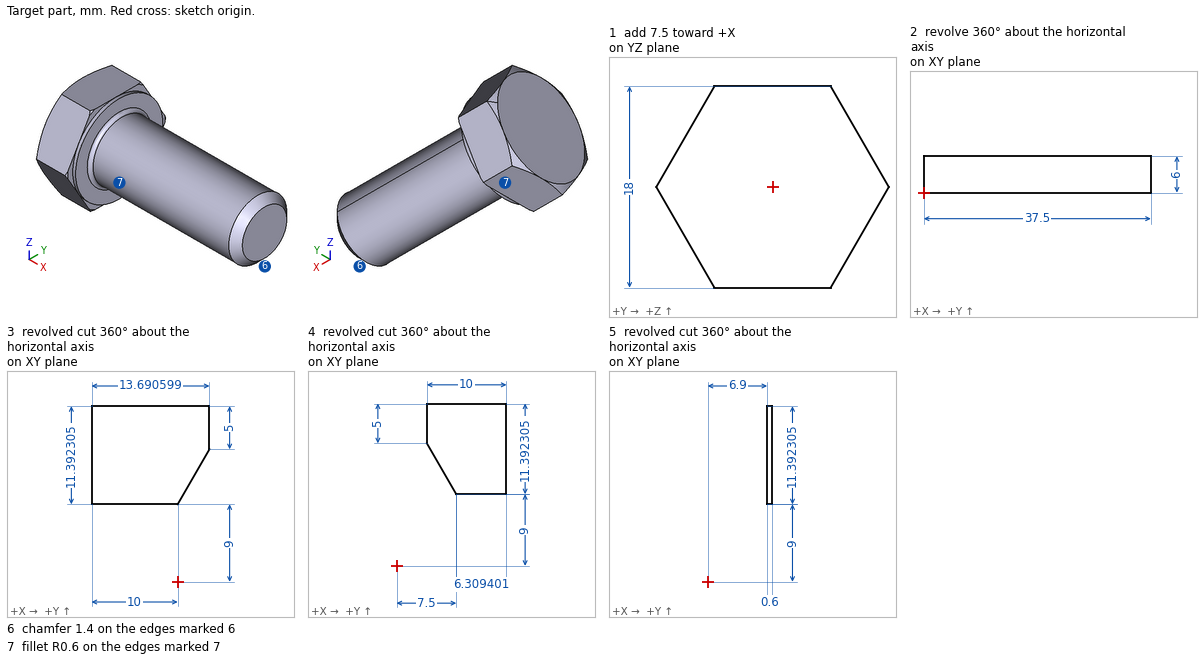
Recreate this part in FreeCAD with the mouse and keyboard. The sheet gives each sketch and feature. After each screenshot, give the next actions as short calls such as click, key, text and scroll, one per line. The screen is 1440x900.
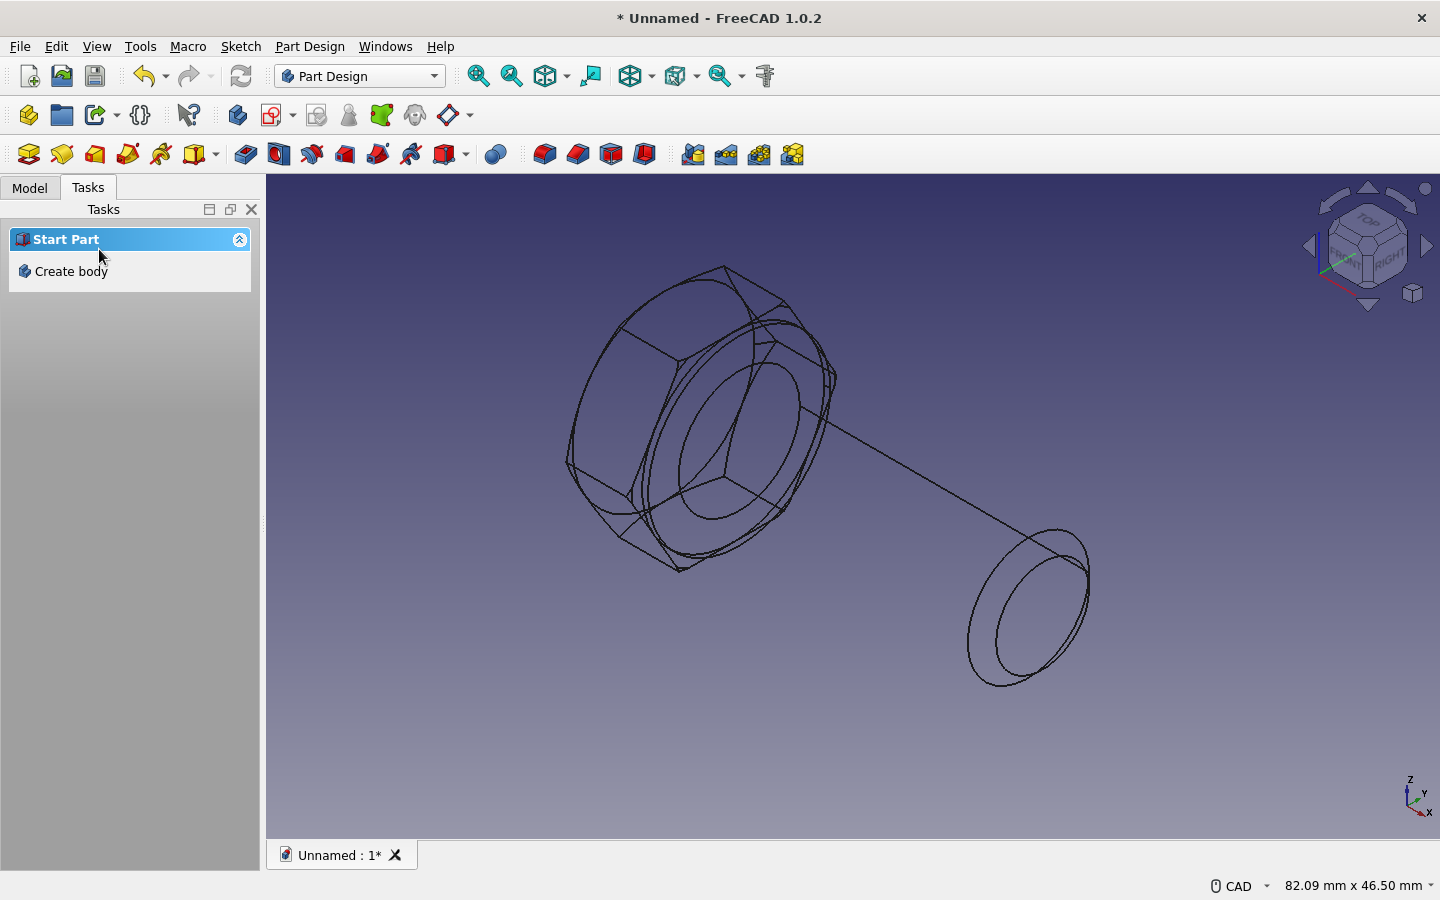
click(679, 475)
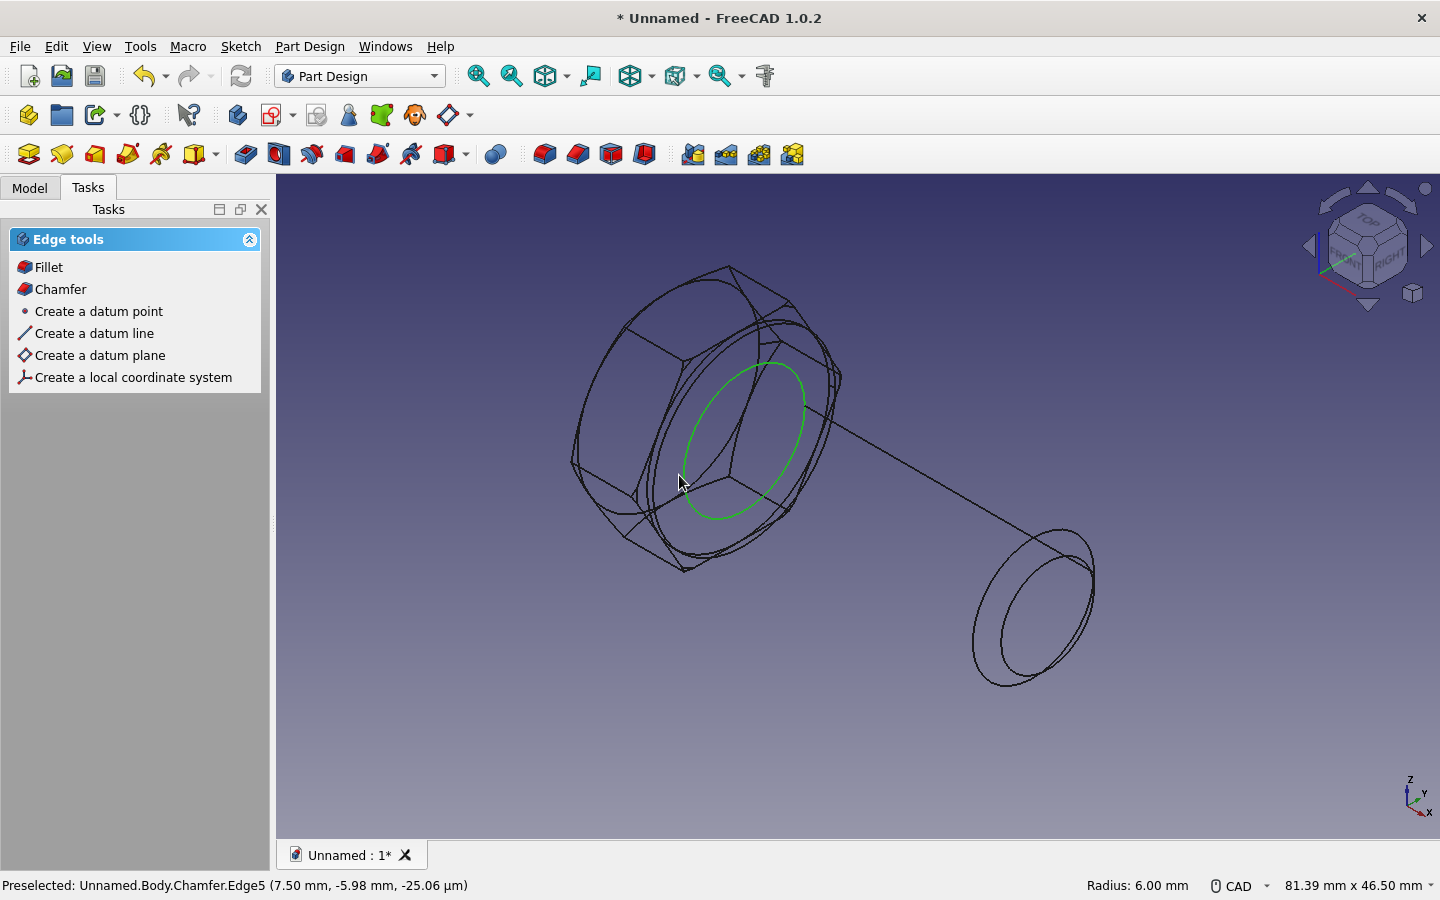
key(v)
key(1)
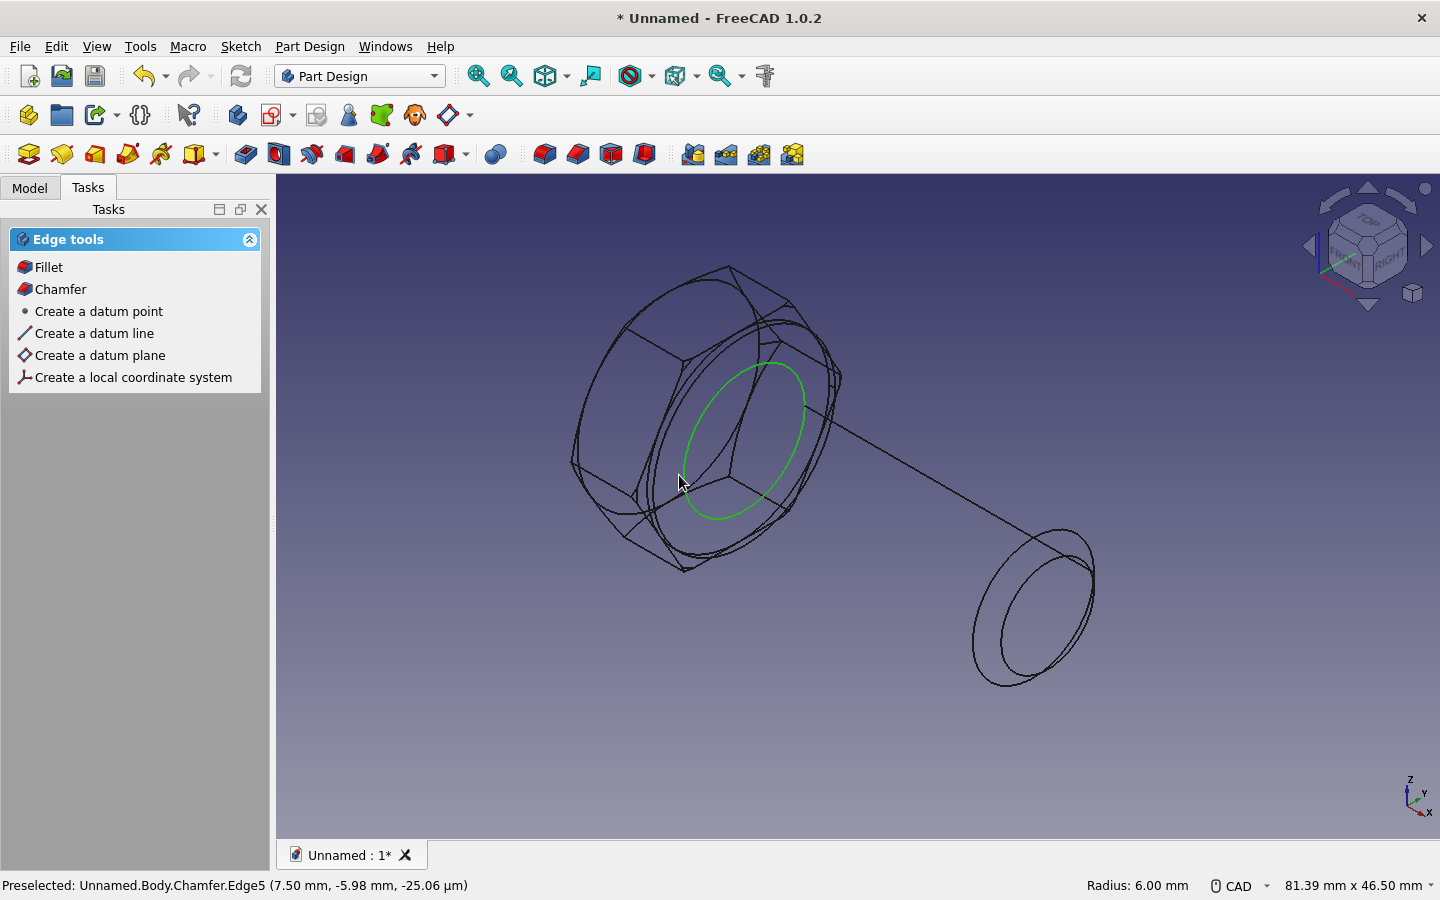
click(545, 154)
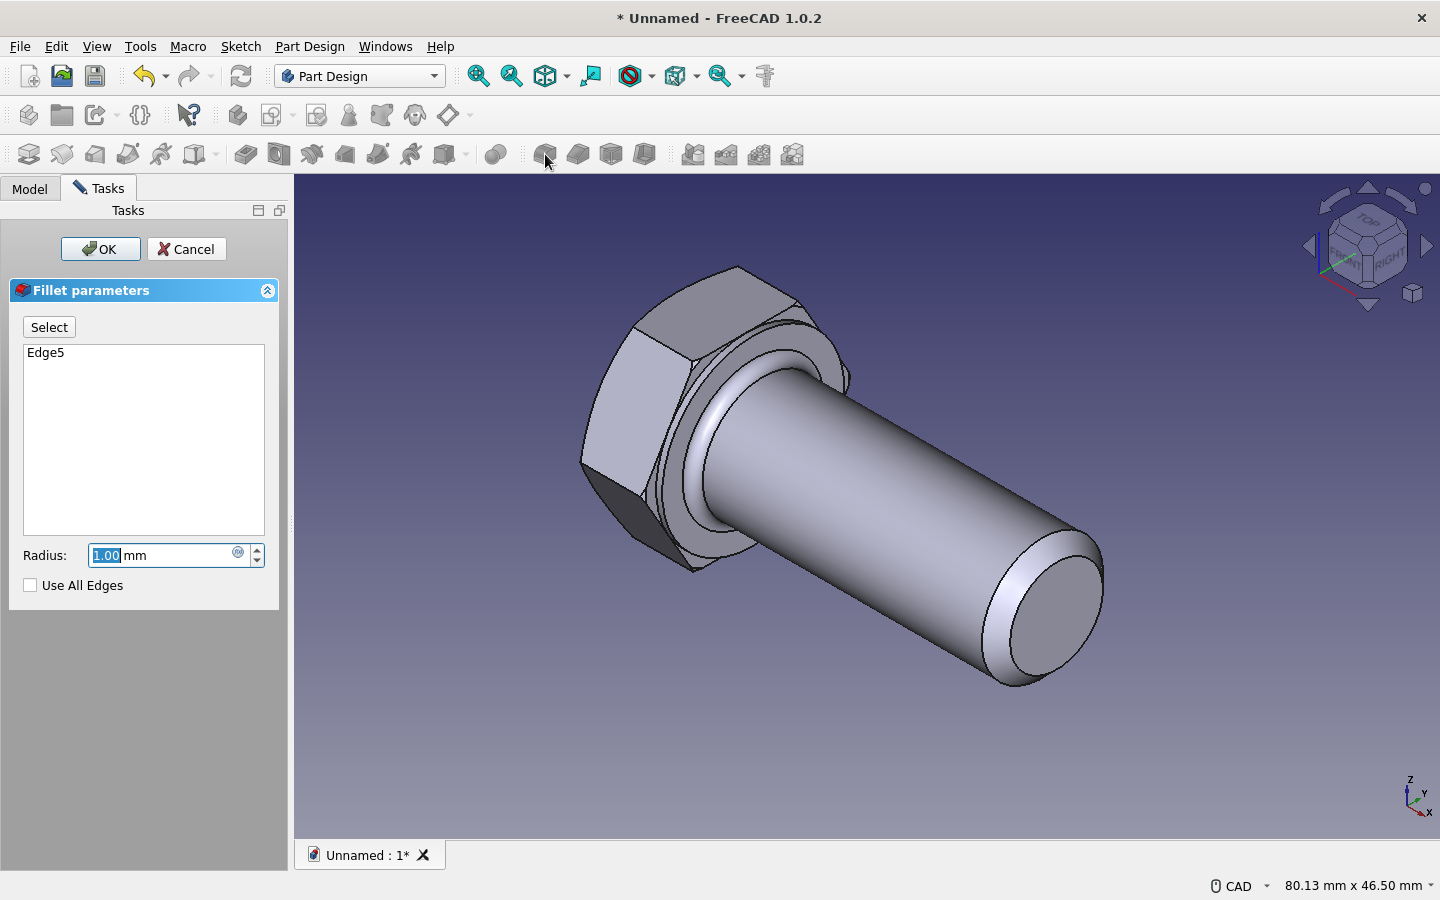
text(0.6)
key(Tab)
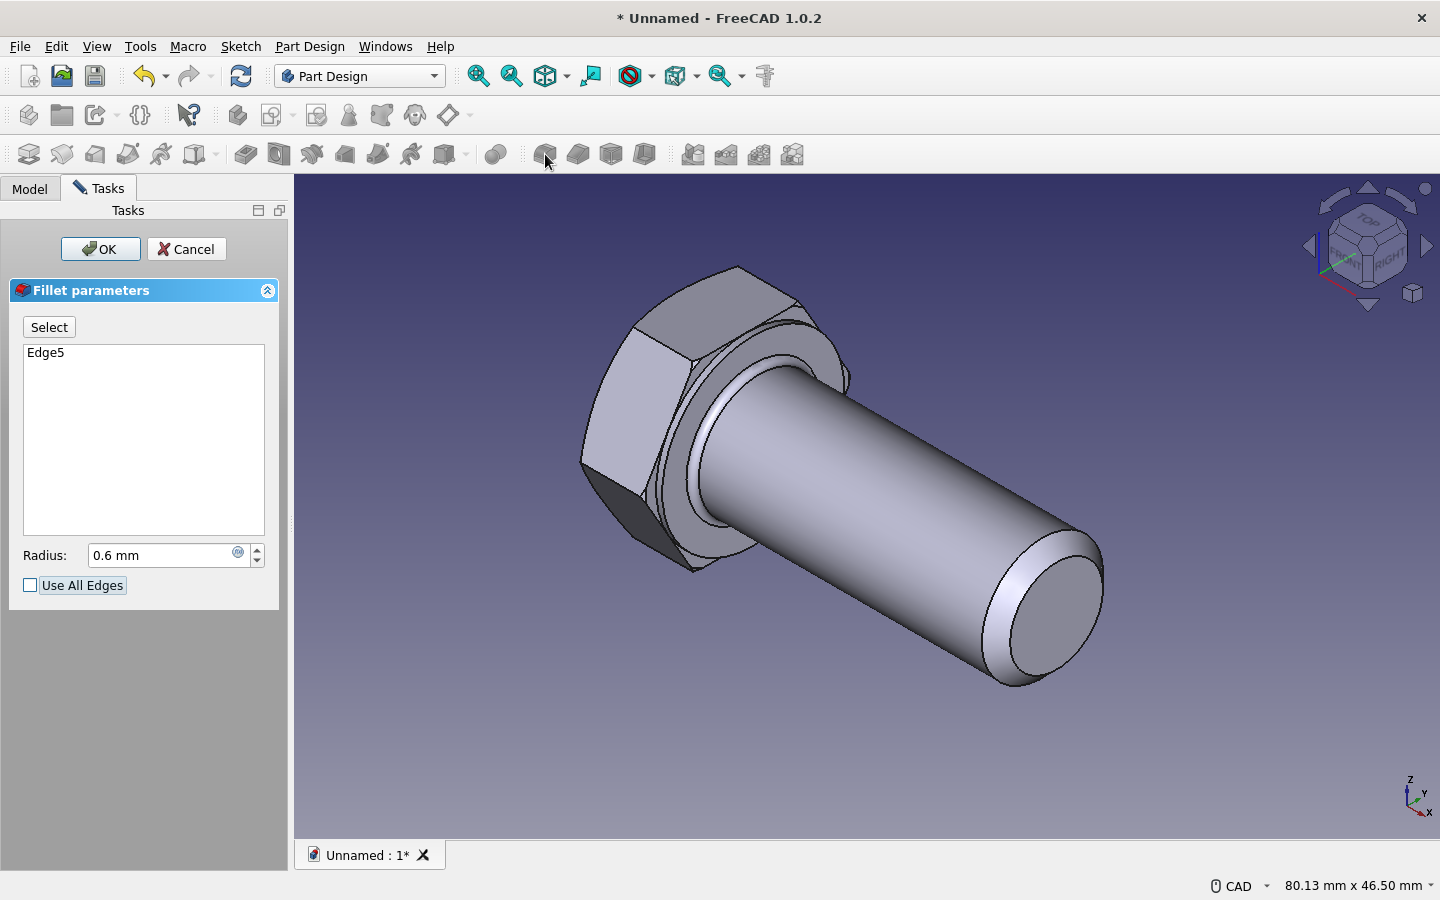
click(101, 249)